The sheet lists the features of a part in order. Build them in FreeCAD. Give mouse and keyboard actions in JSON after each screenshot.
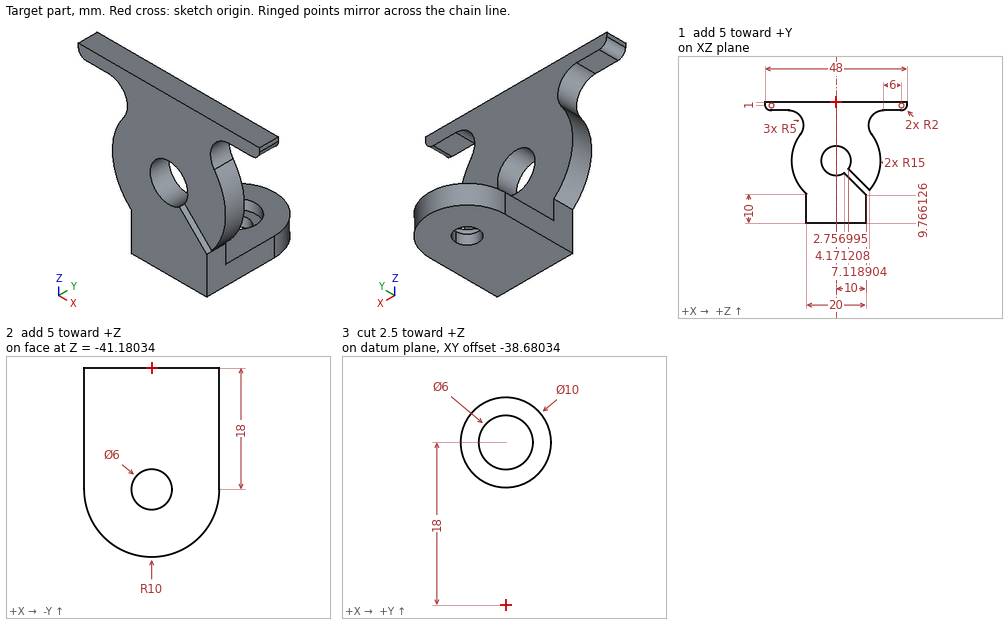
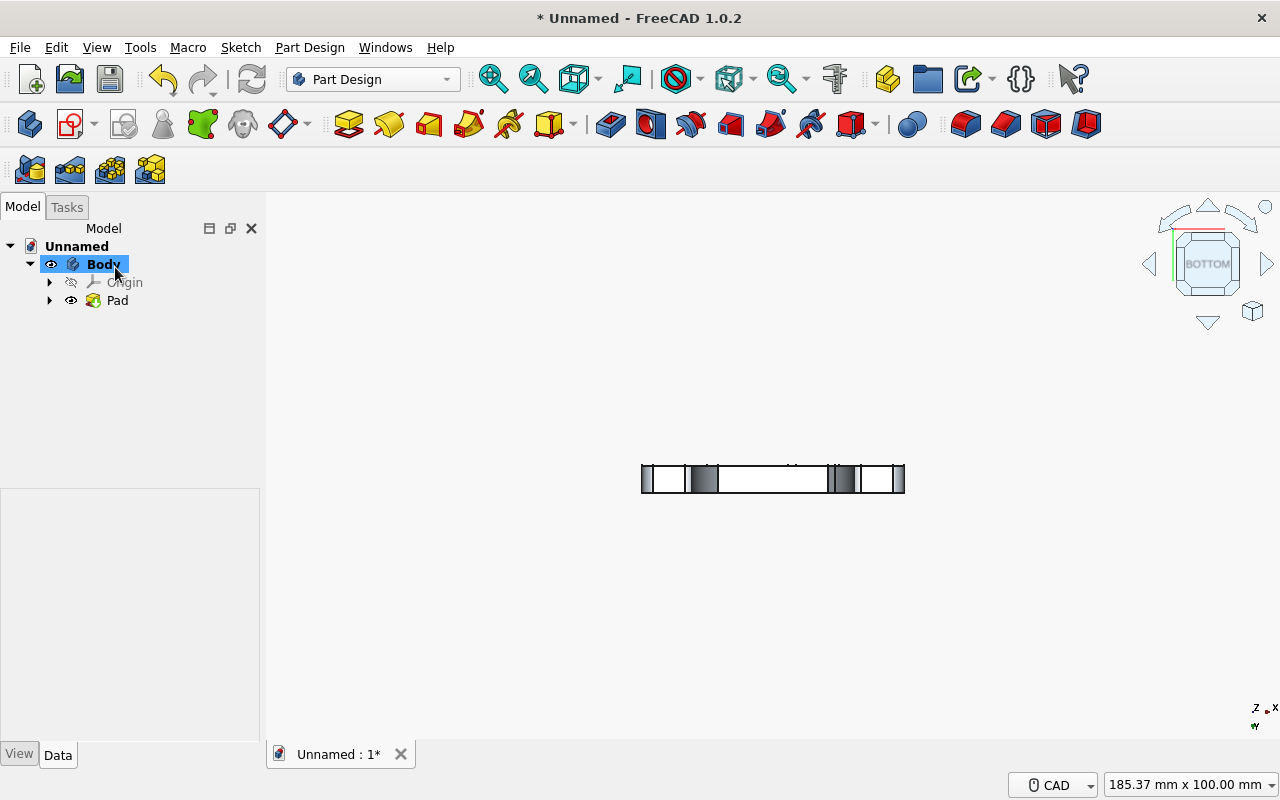
{"action": "left_click", "coordinate": [494, 80]}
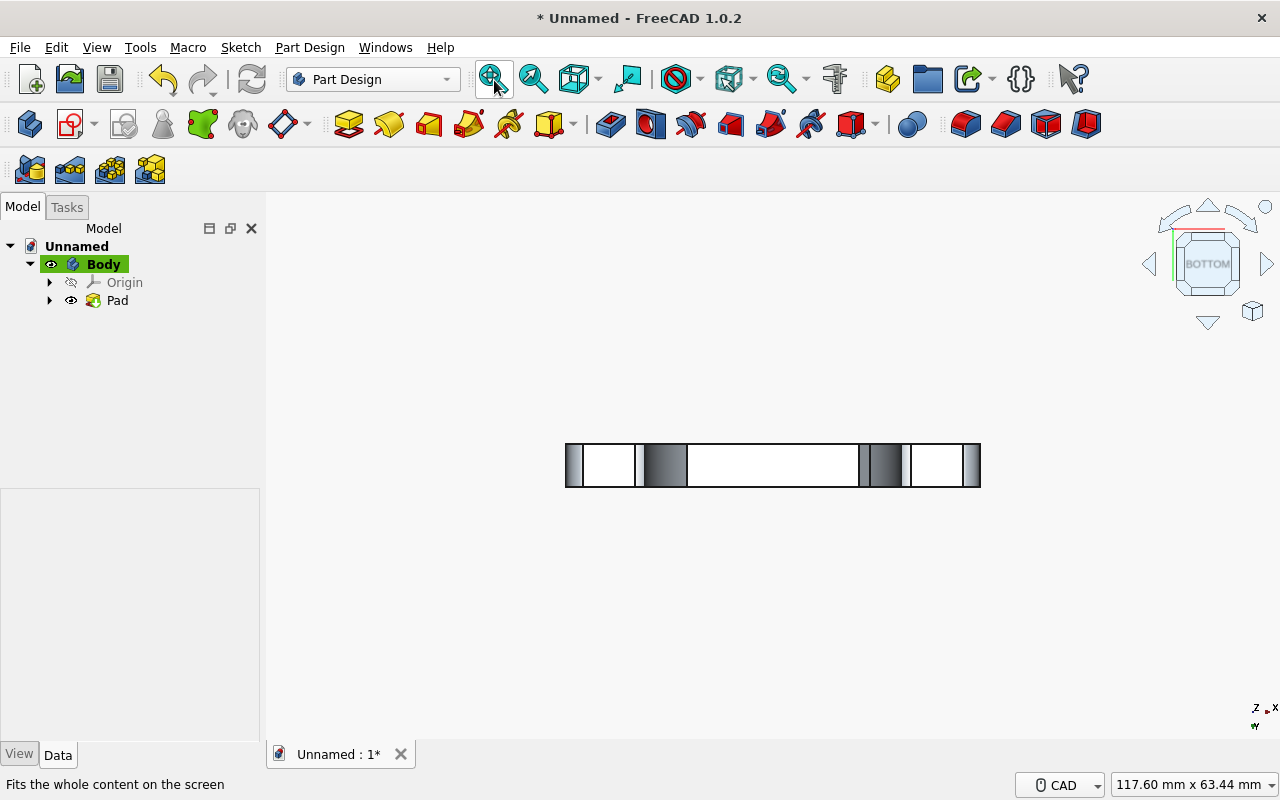
{"action": "left_click", "coordinate": [822, 464]}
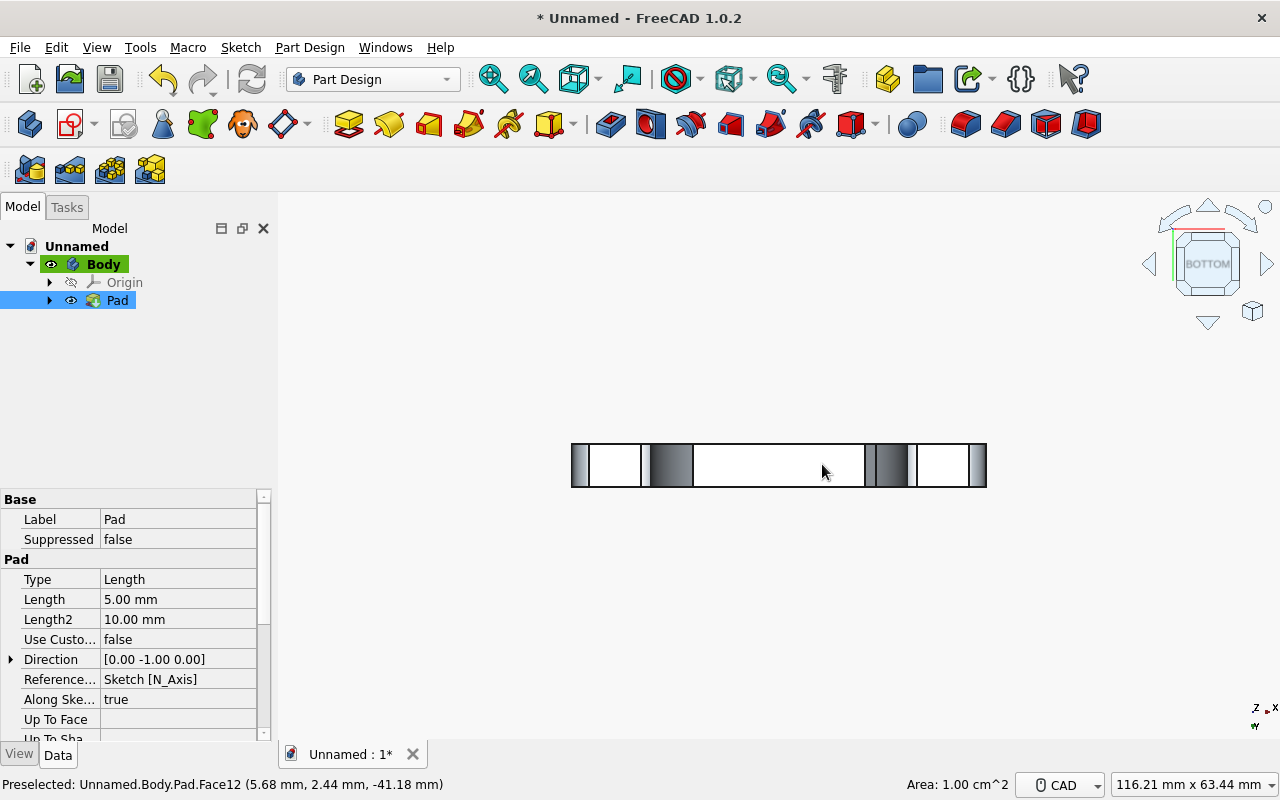
{"action": "left_click", "coordinate": [70, 124]}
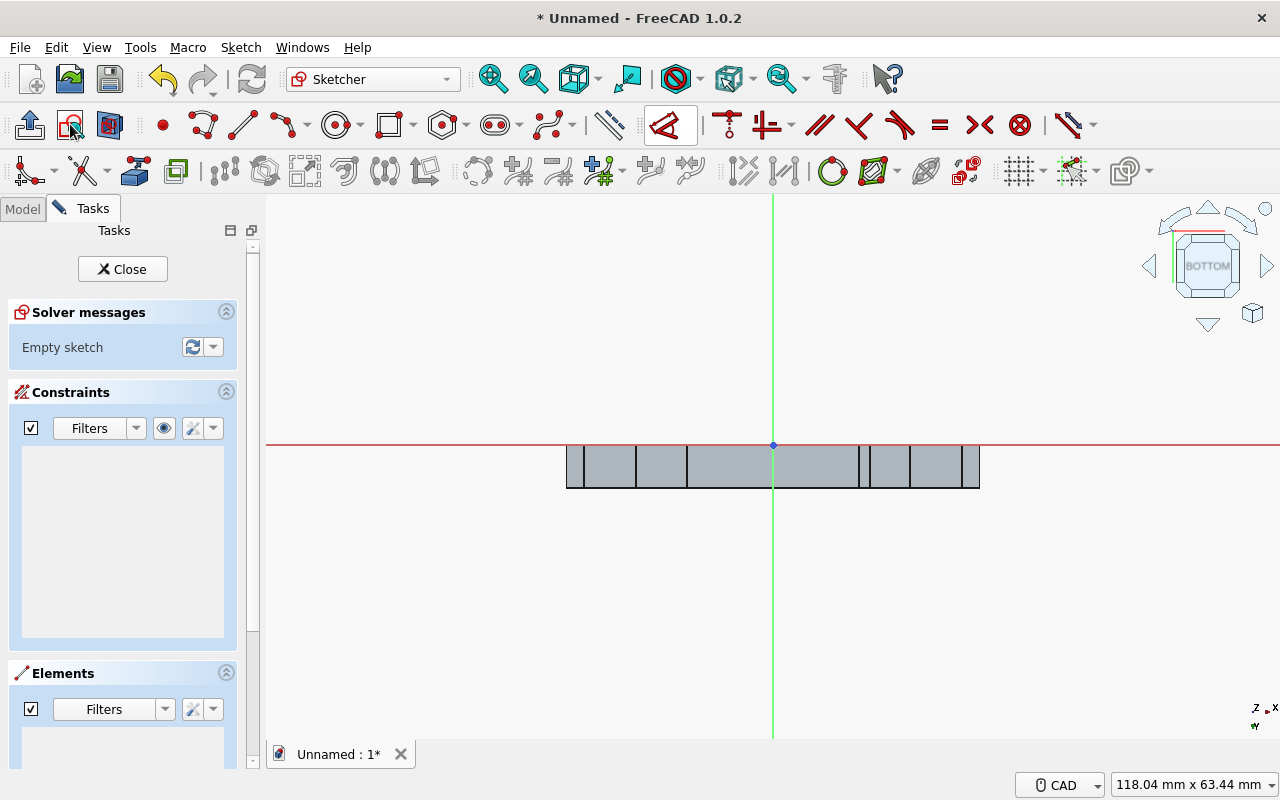
{"action": "scroll", "coordinate": [912, 711], "scroll_direction": "up", "scroll_amount": 2}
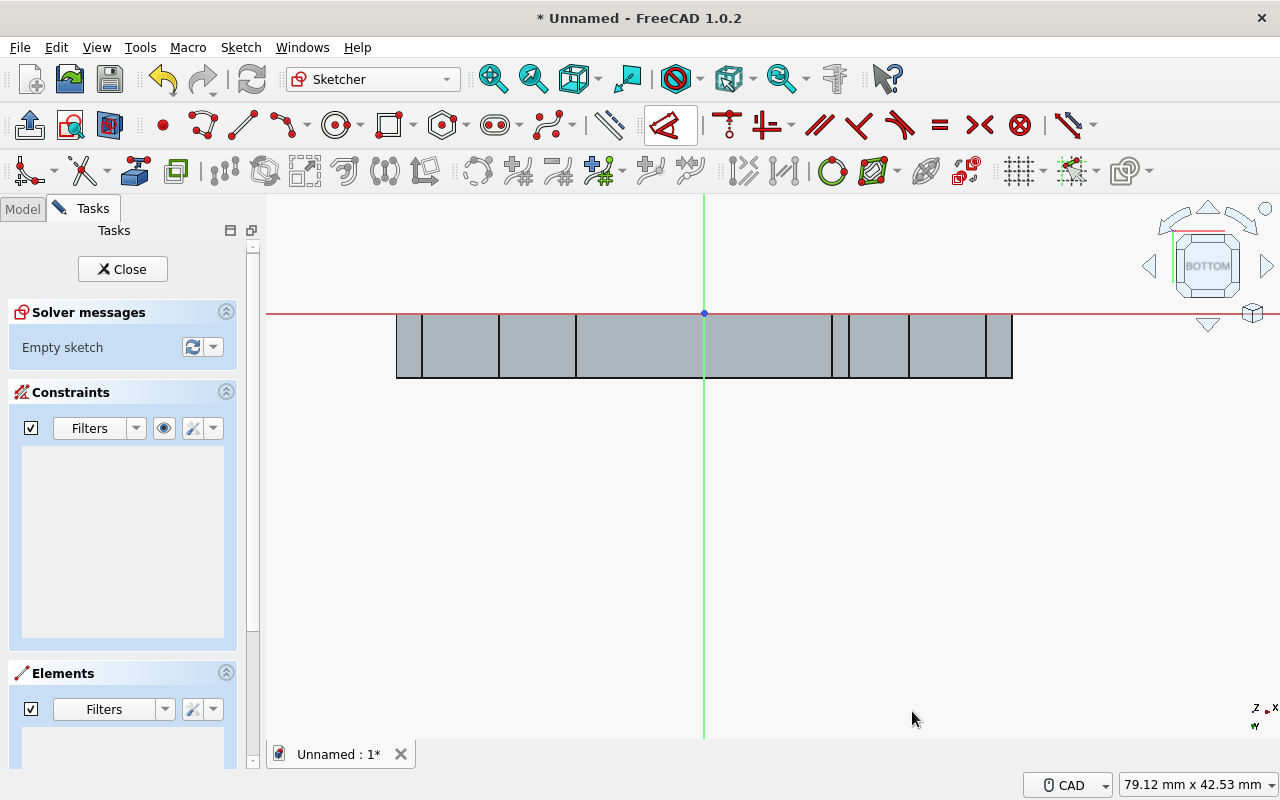
{"action": "left_click", "coordinate": [204, 126]}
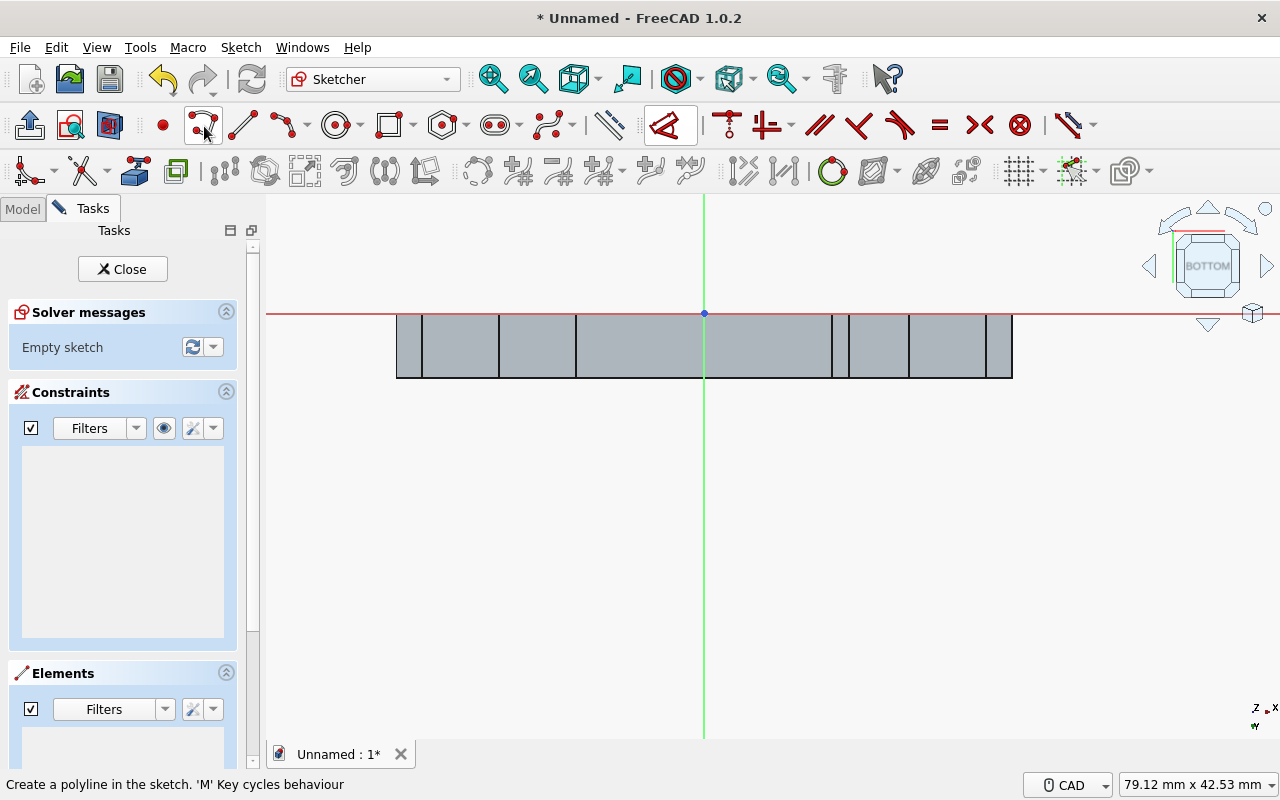
{"action": "left_click", "coordinate": [832, 544]}
{"action": "left_click", "coordinate": [832, 314]}
{"action": "left_click", "coordinate": [576, 323]}
{"action": "left_click", "coordinate": [576, 544]}
{"action": "right_click", "coordinate": [576, 544]}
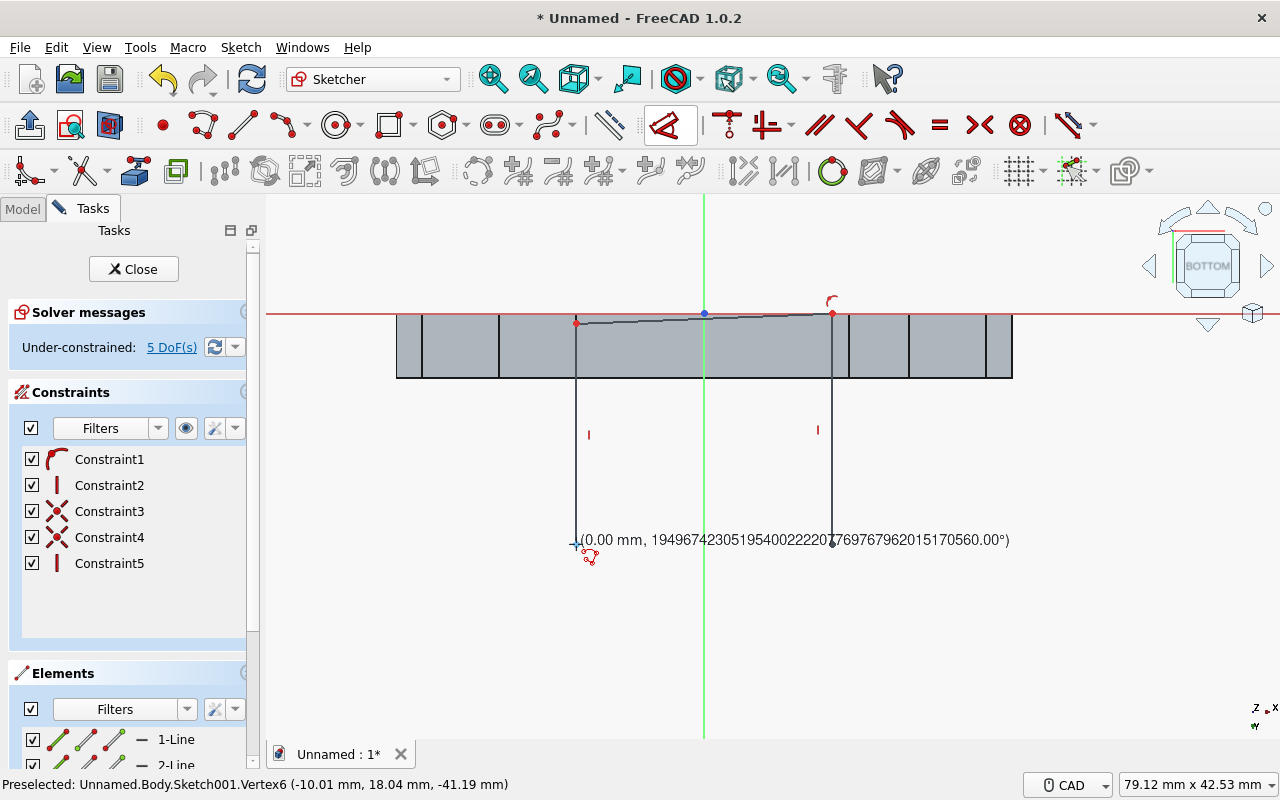
{"action": "left_click", "coordinate": [284, 126]}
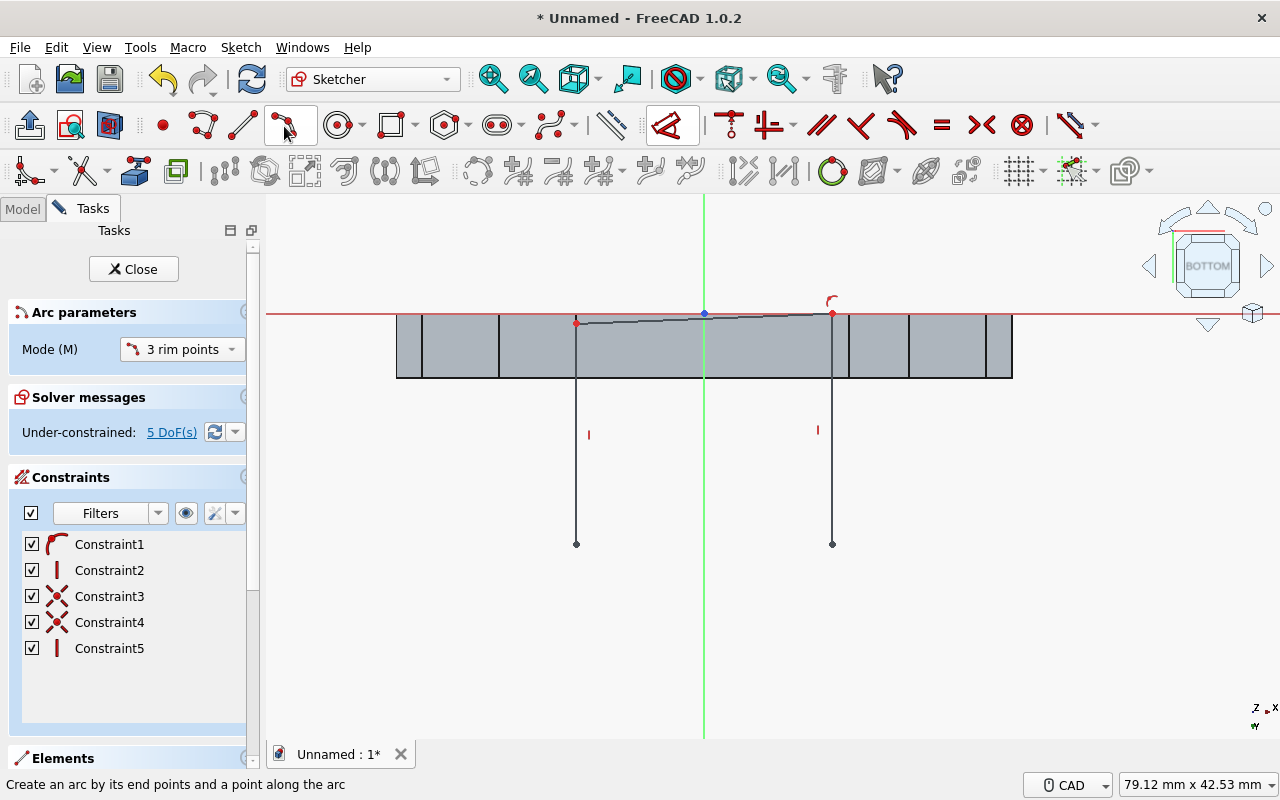
{"action": "left_click", "coordinate": [576, 545]}
{"action": "left_click", "coordinate": [832, 545]}
{"action": "left_click", "coordinate": [665, 666]}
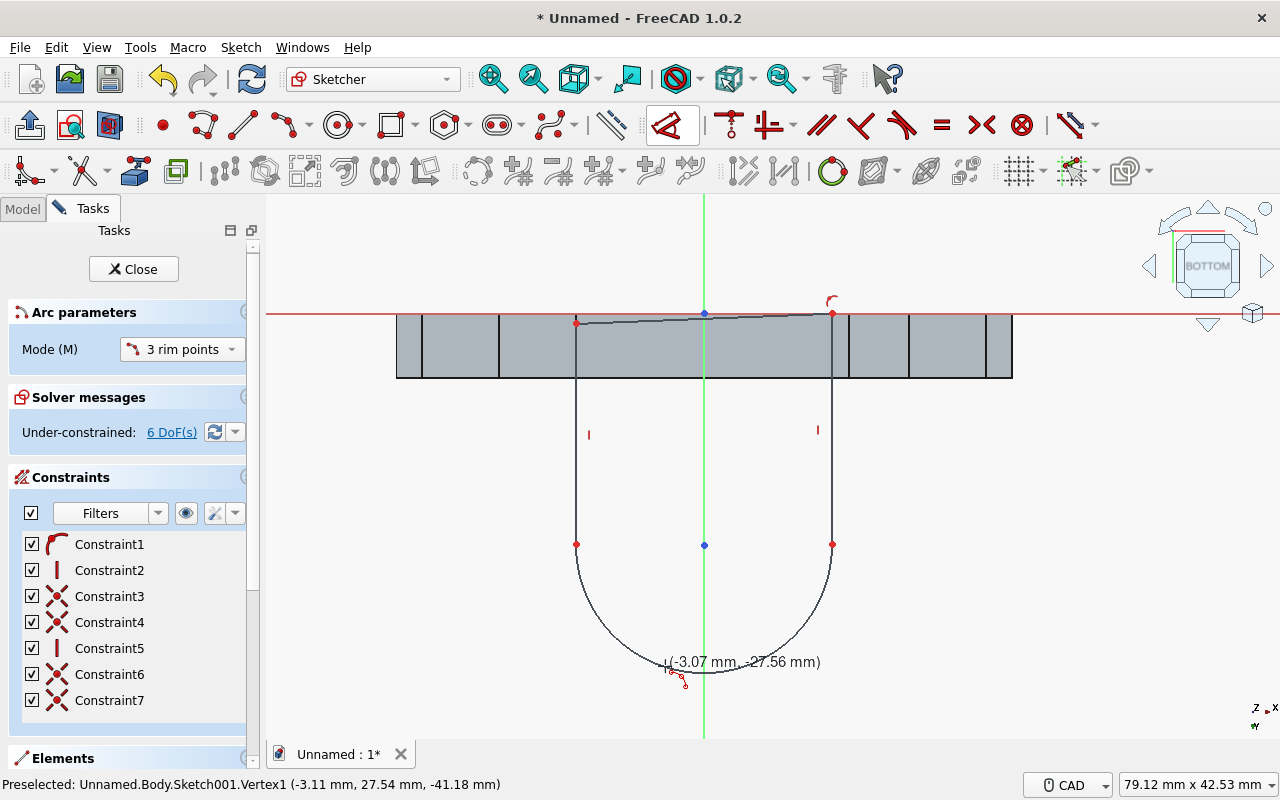
{"action": "key", "text": "g c"}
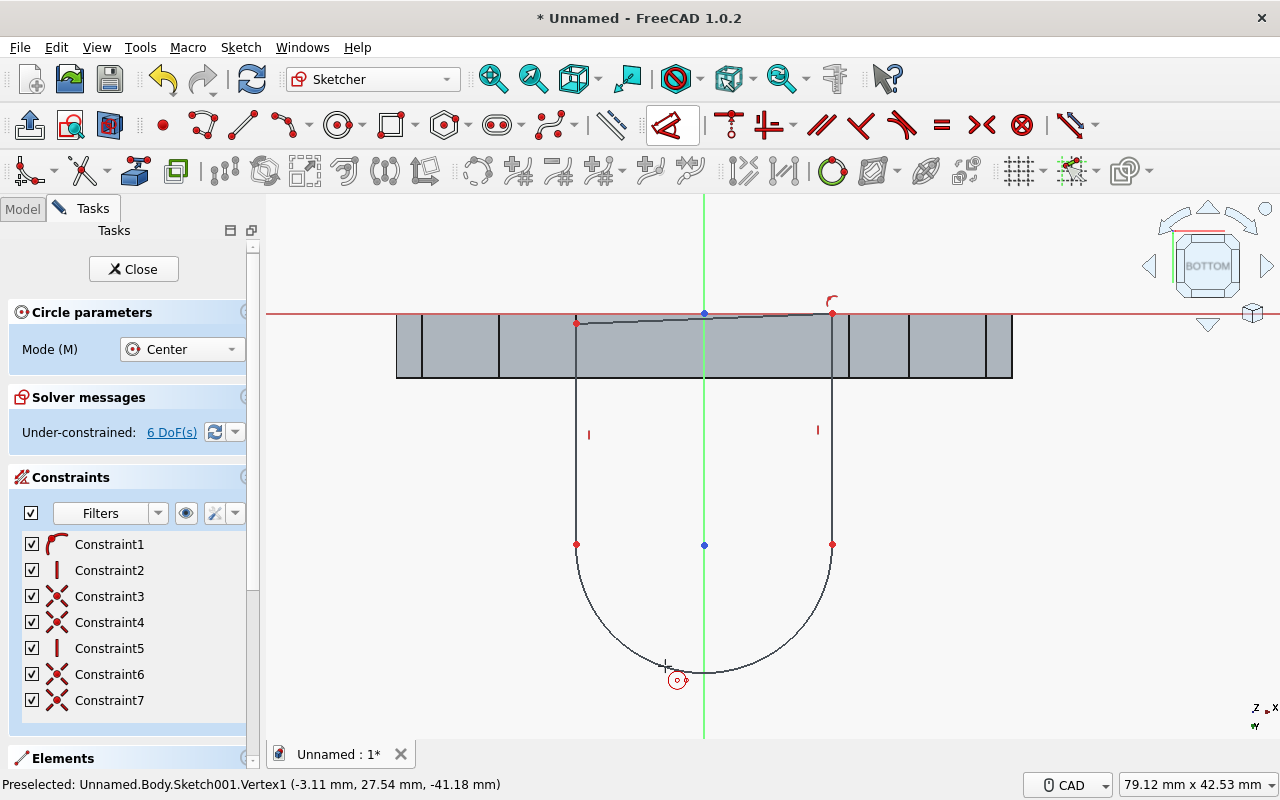
{"action": "left_click", "coordinate": [704, 544]}
{"action": "left_click", "coordinate": [732, 517]}
{"action": "key", "text": "Escape"}